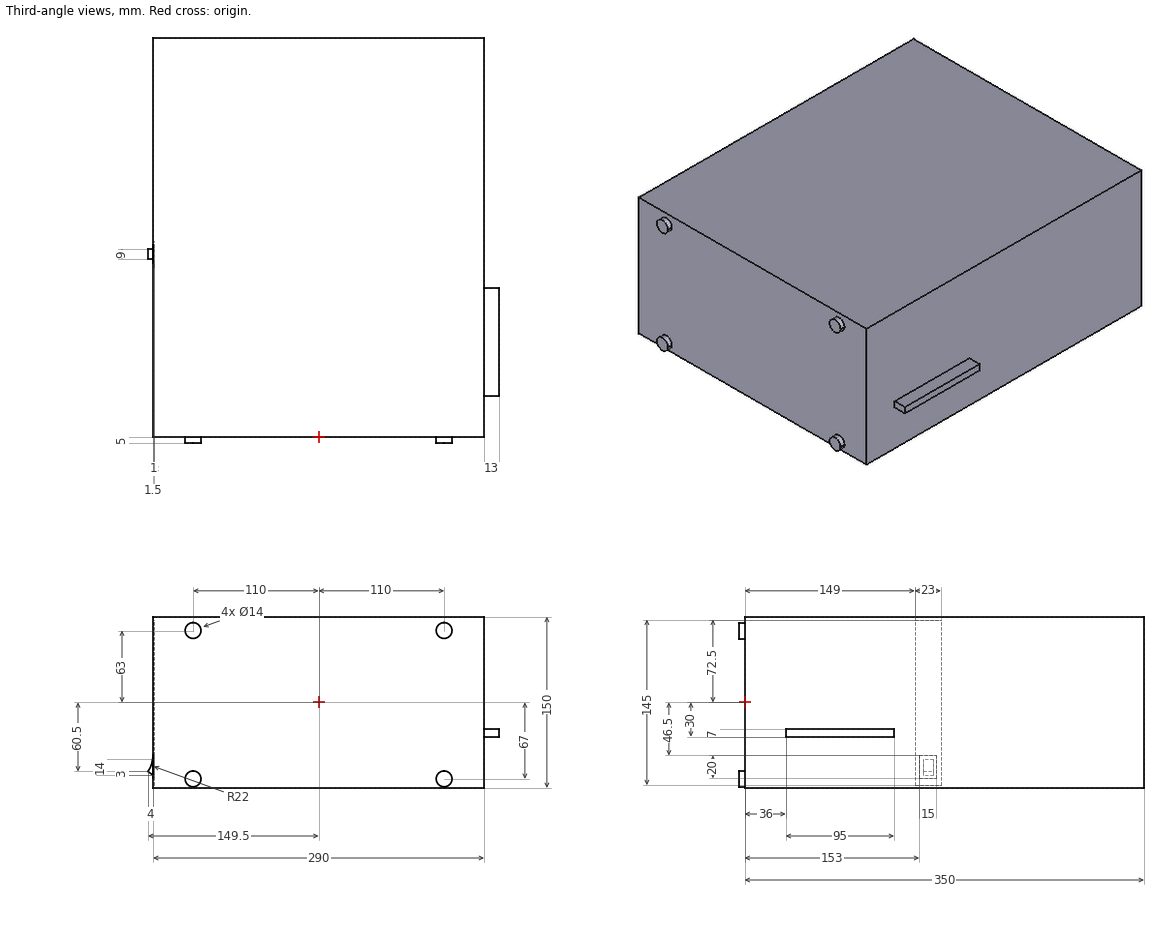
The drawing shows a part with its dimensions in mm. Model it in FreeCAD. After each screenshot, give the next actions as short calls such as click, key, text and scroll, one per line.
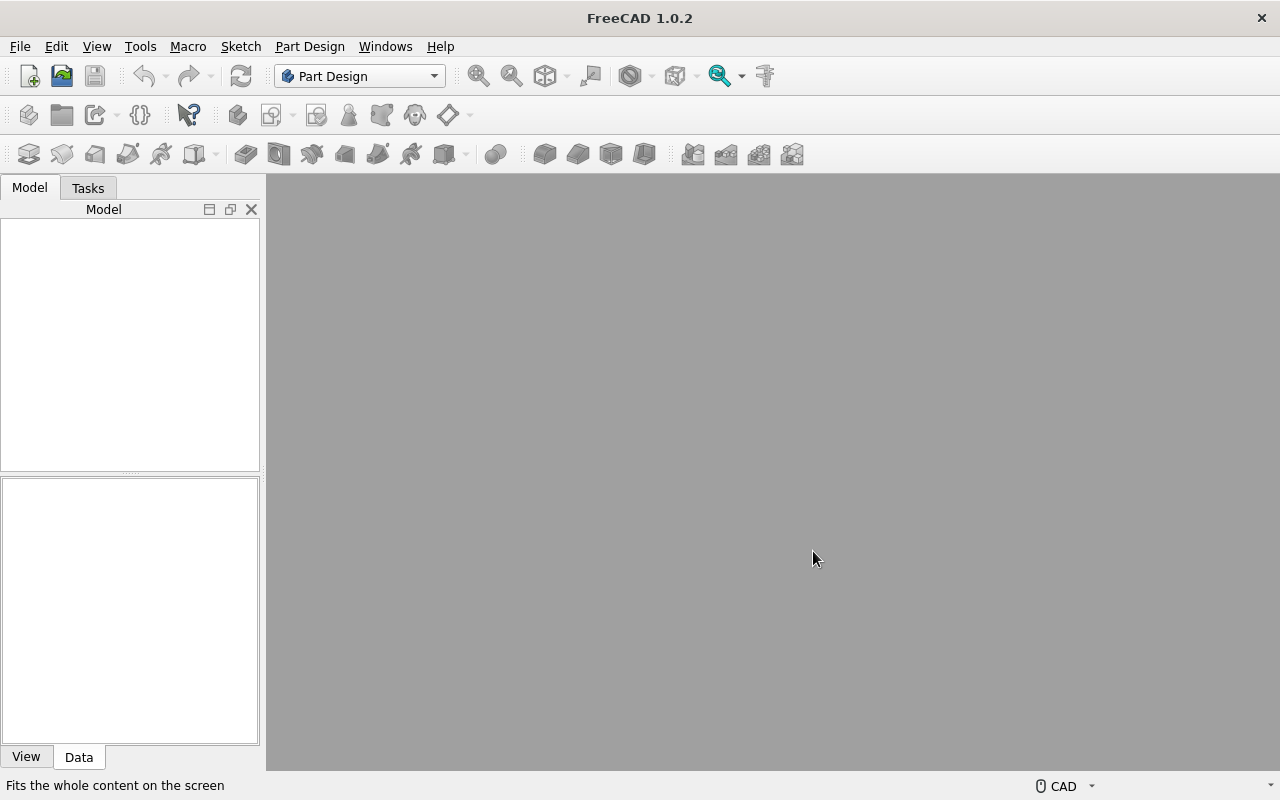
click(29, 76)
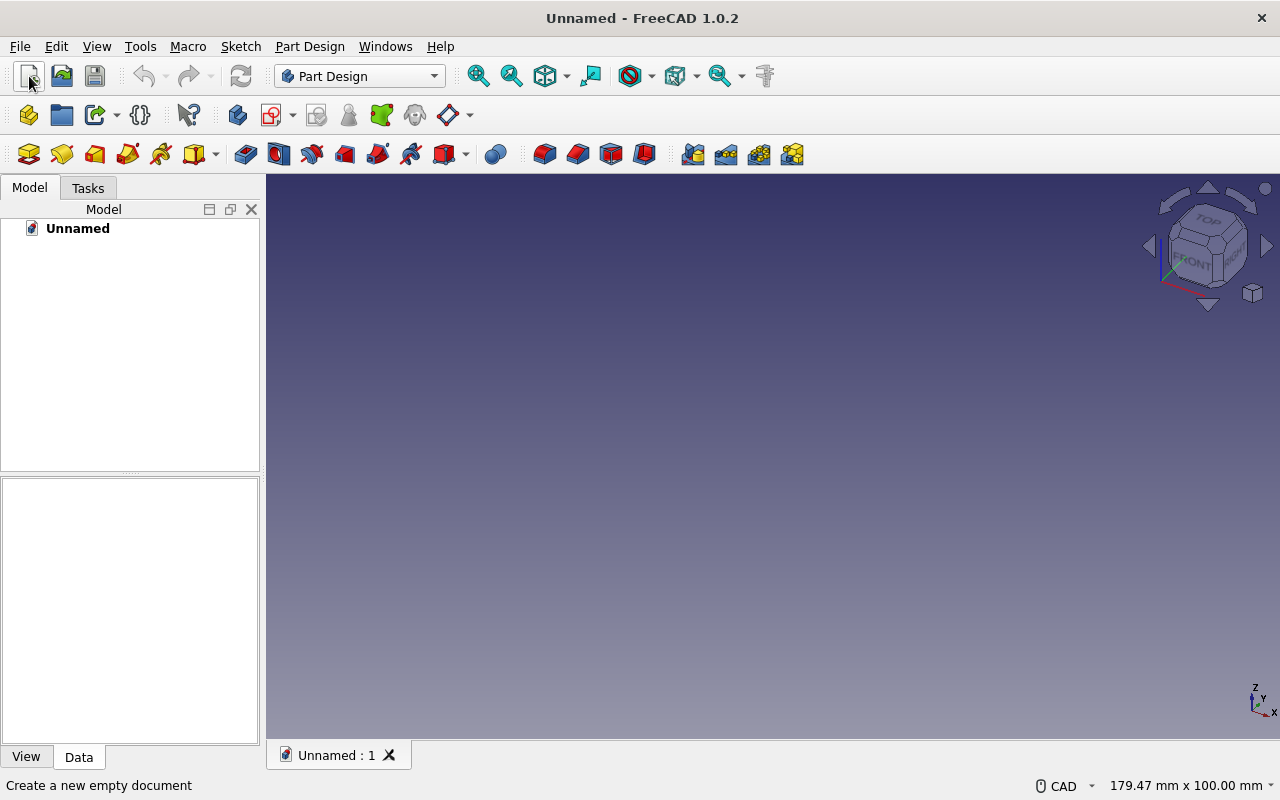
click(270, 116)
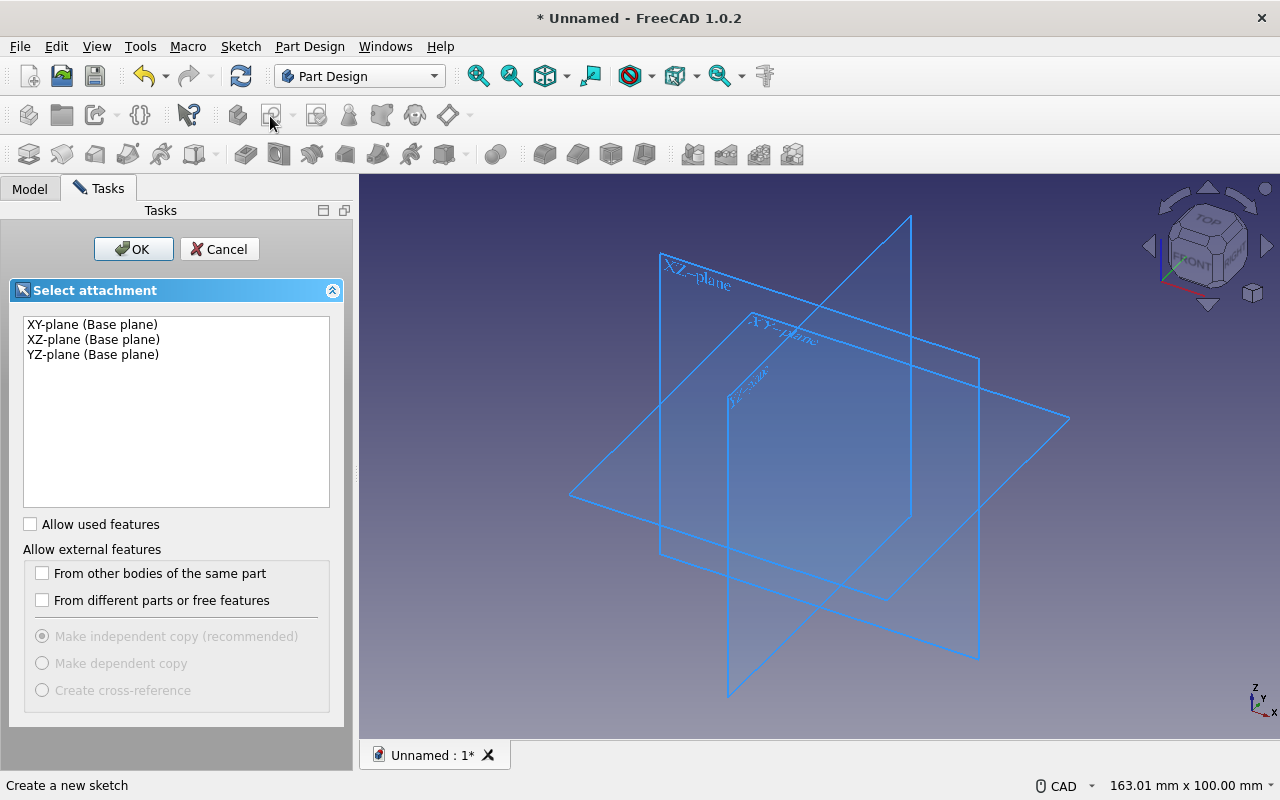
click(84, 340)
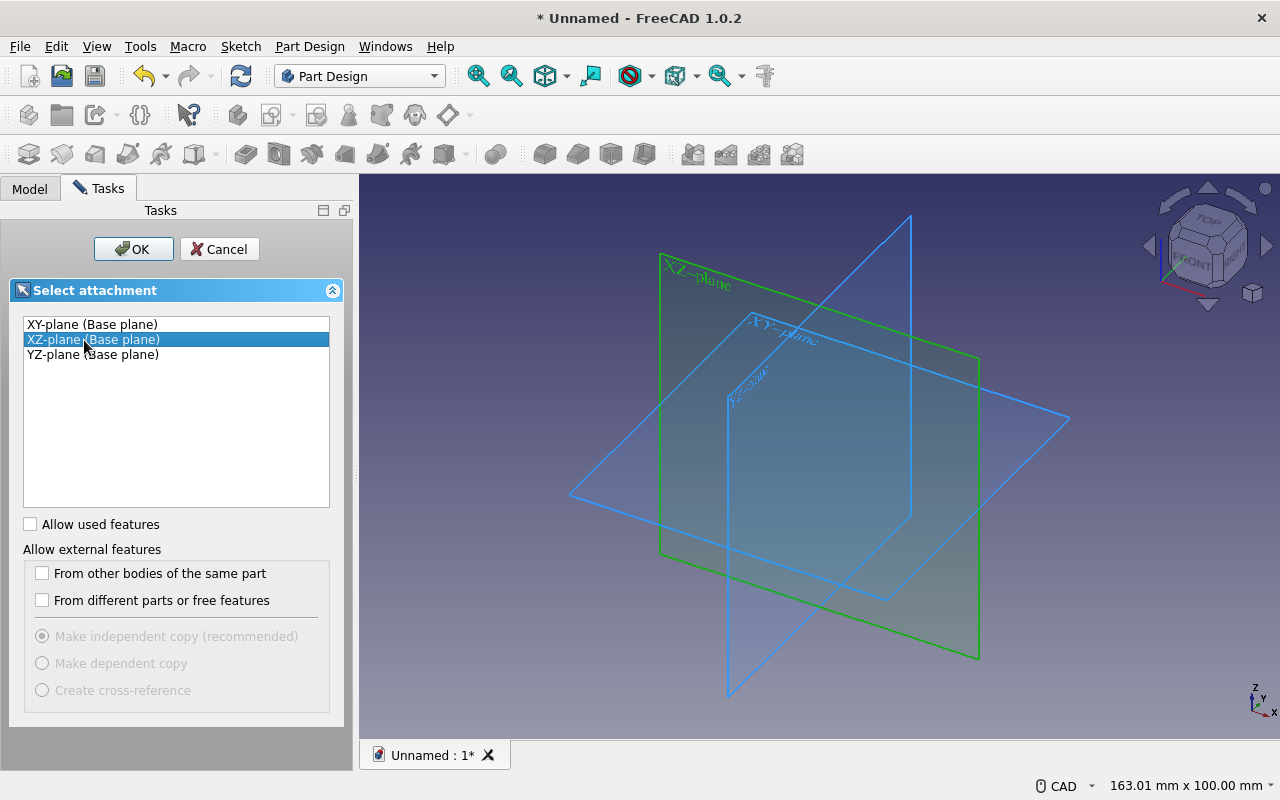
click(134, 249)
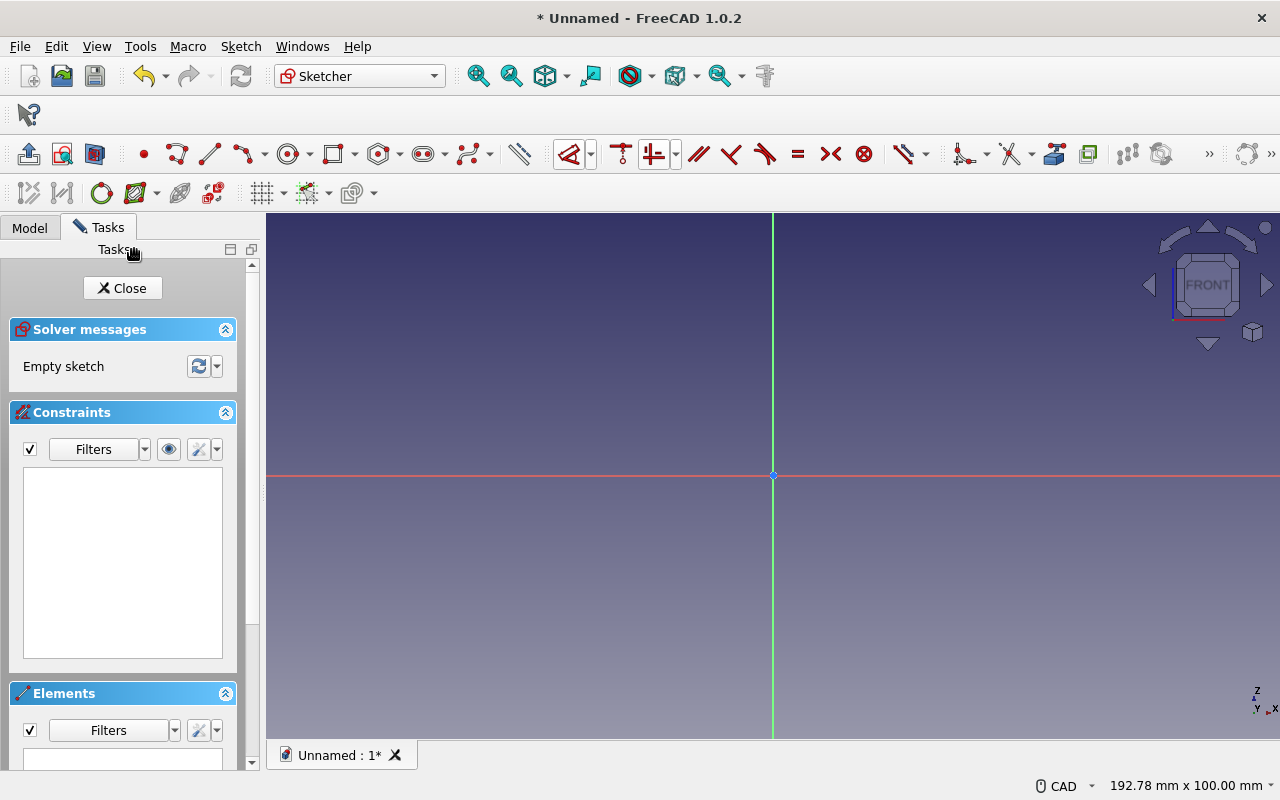
scroll(665, 476, down, 5)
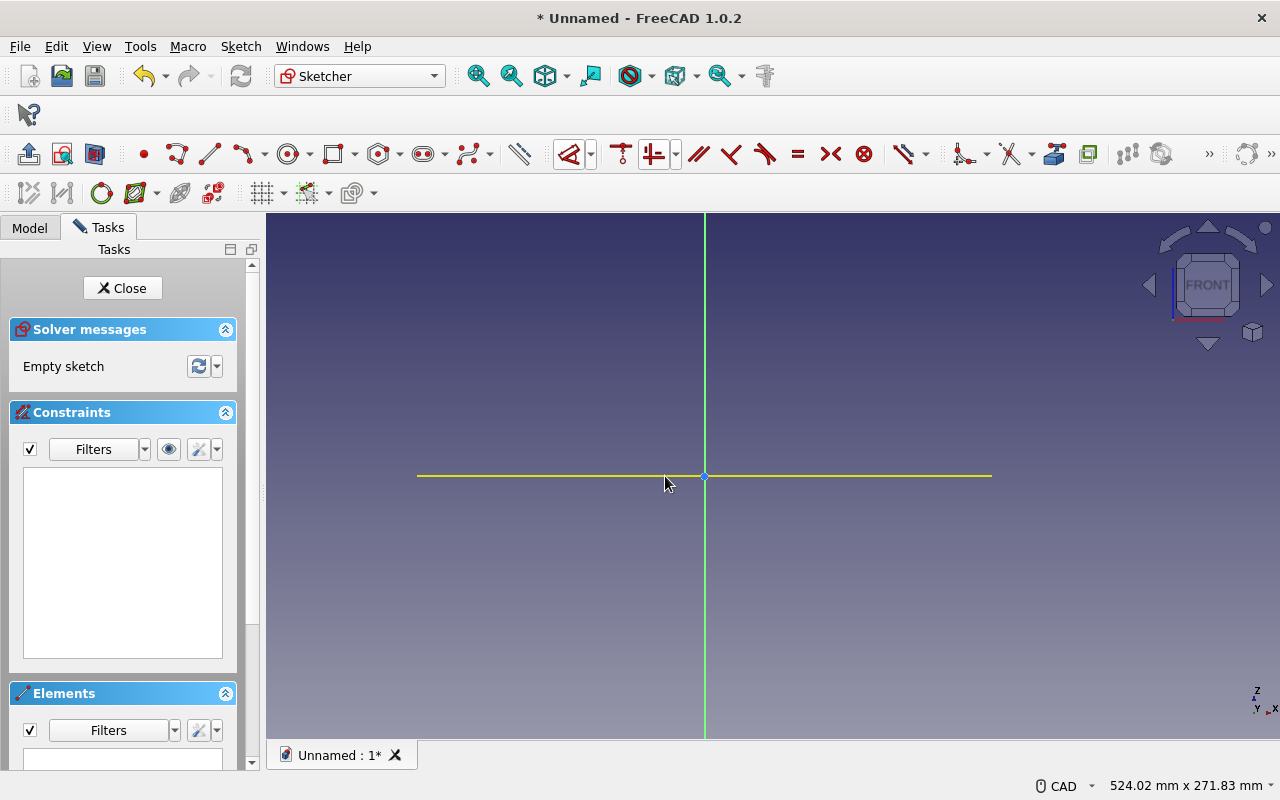
key(g)
key(v)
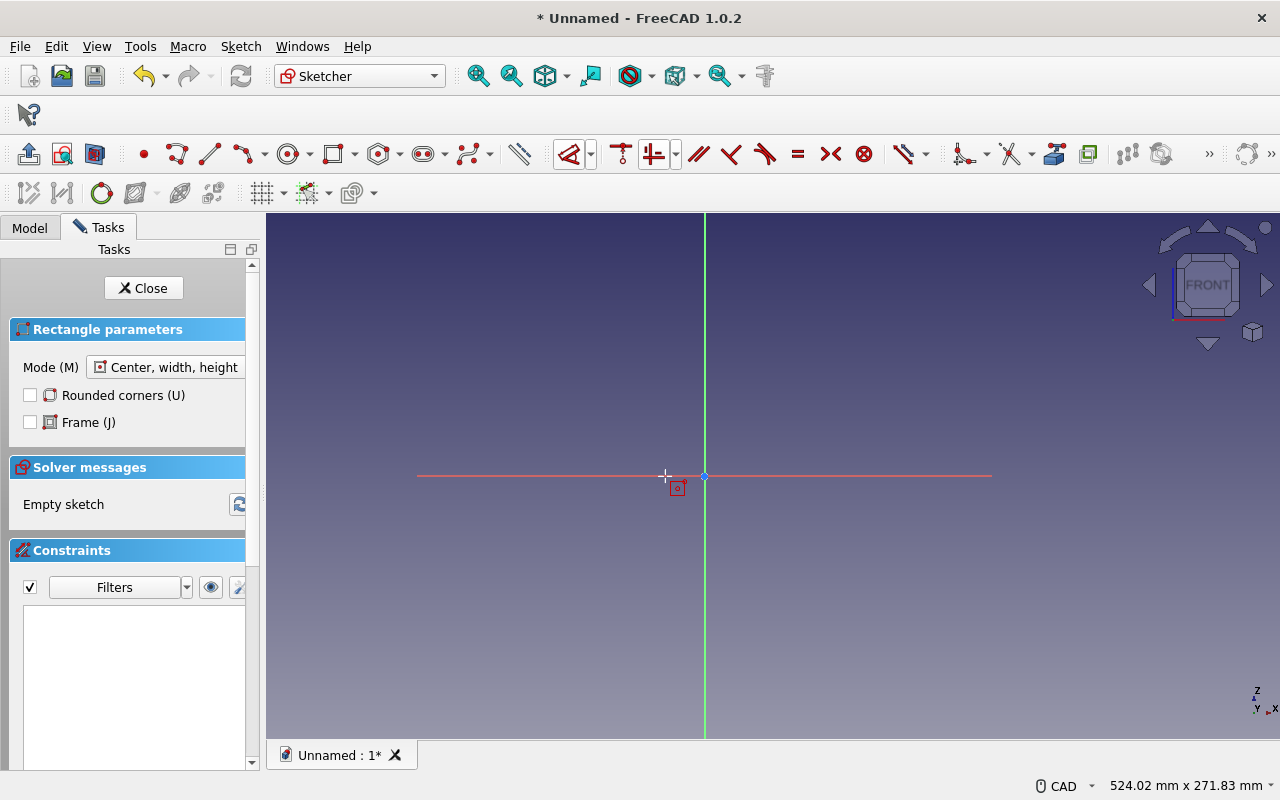
click(705, 476)
click(986, 331)
key(Escape)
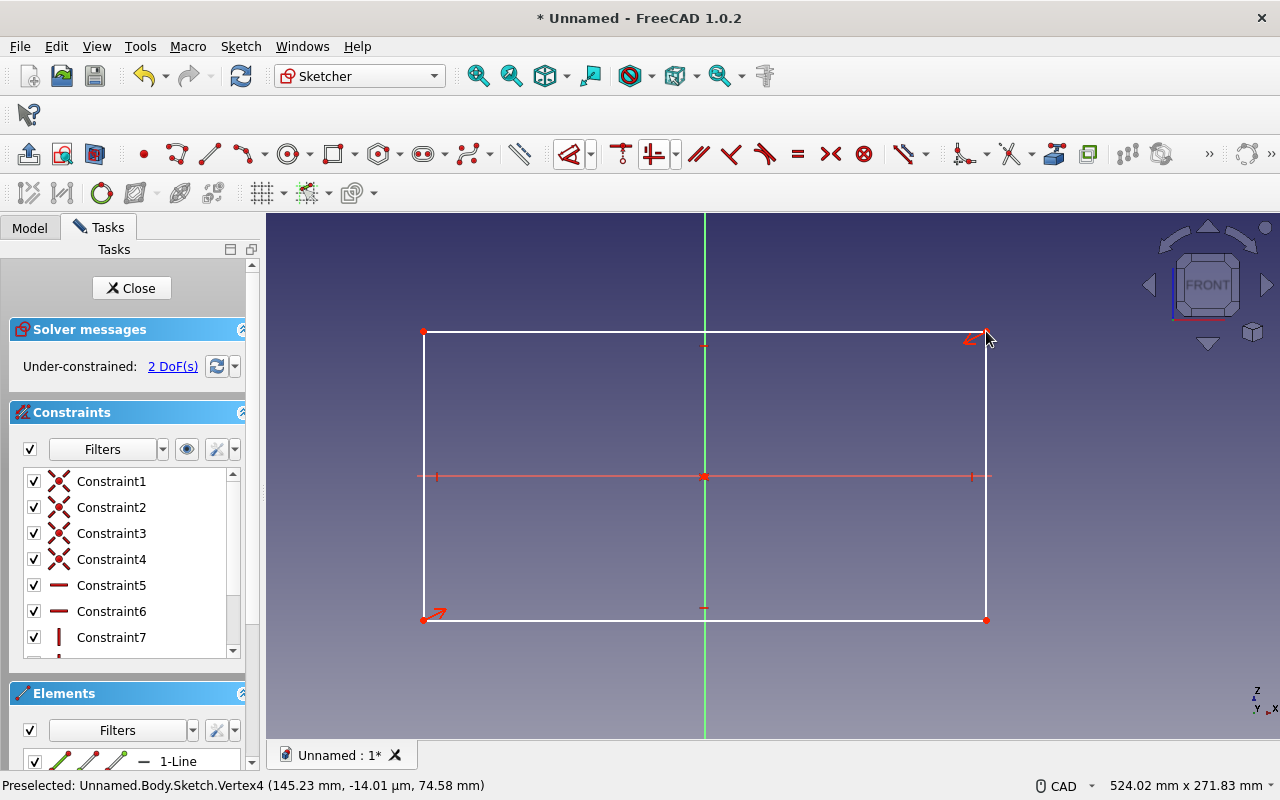
click(568, 154)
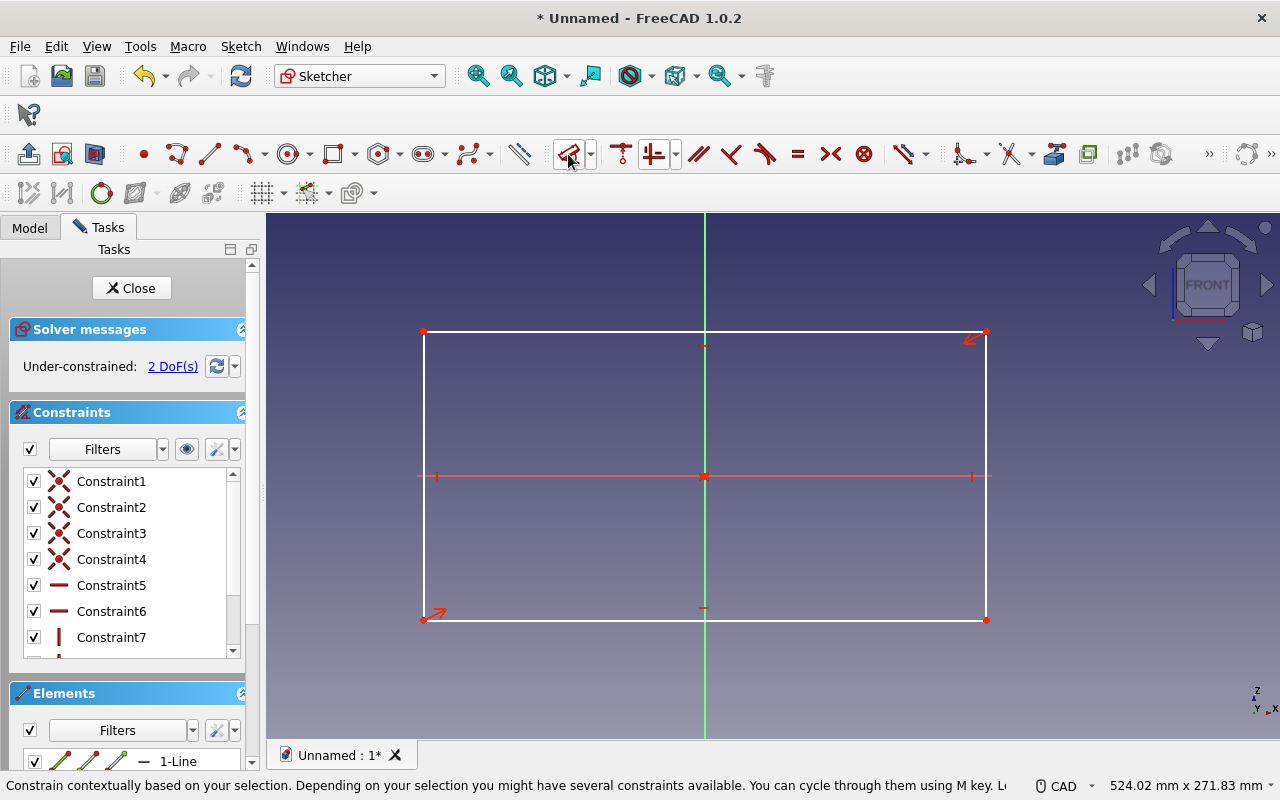
click(593, 621)
click(576, 655)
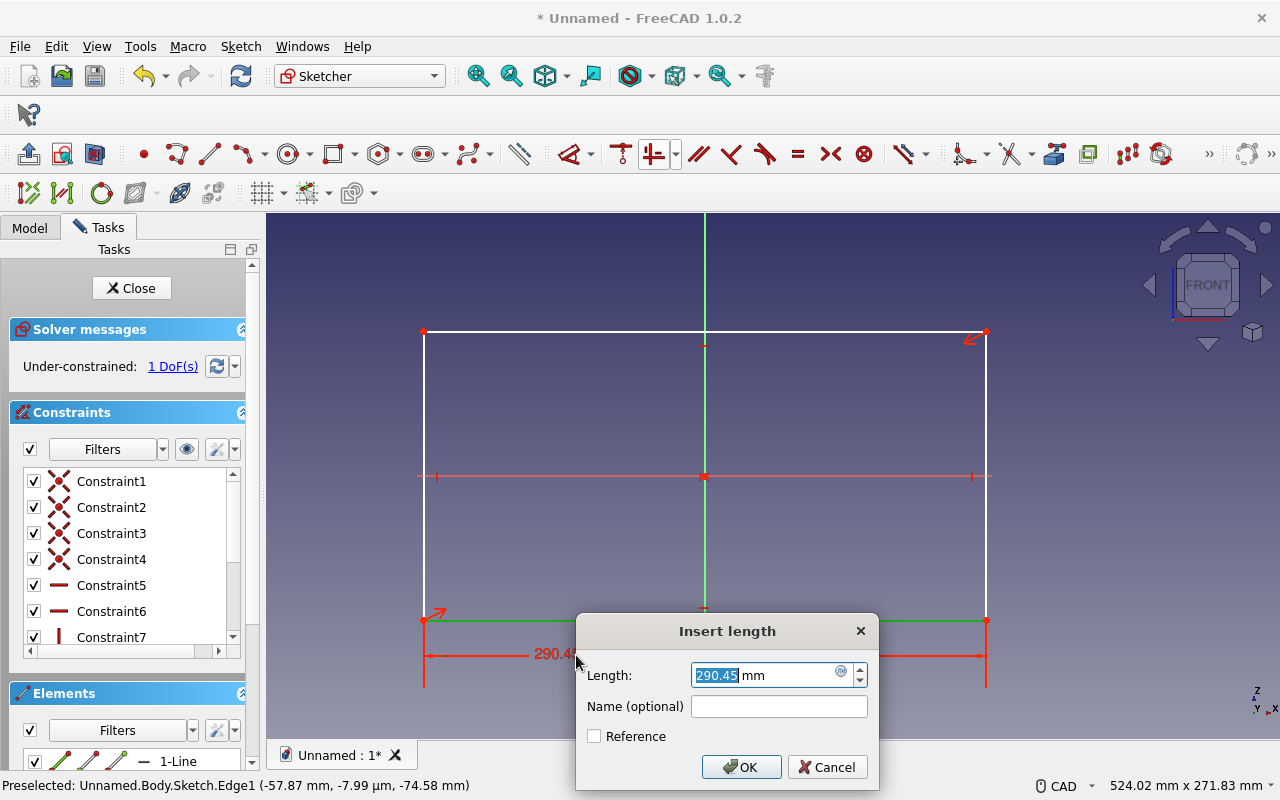
text(290)
key(Return)